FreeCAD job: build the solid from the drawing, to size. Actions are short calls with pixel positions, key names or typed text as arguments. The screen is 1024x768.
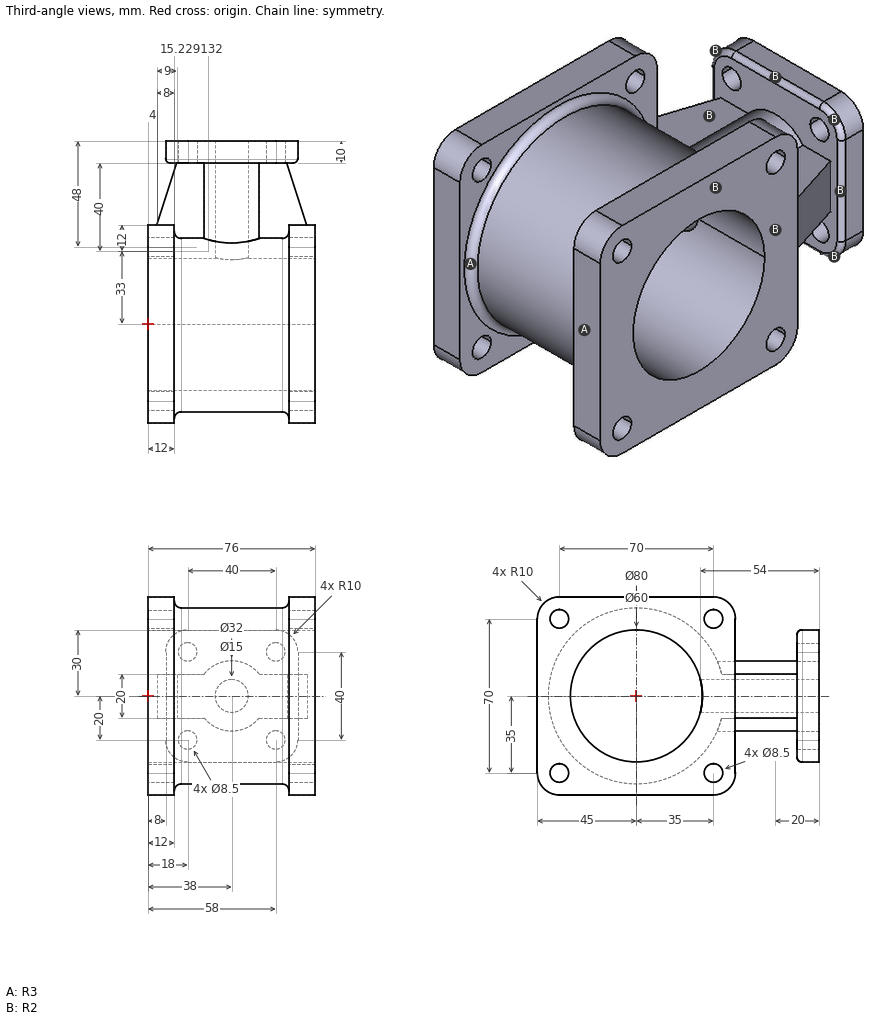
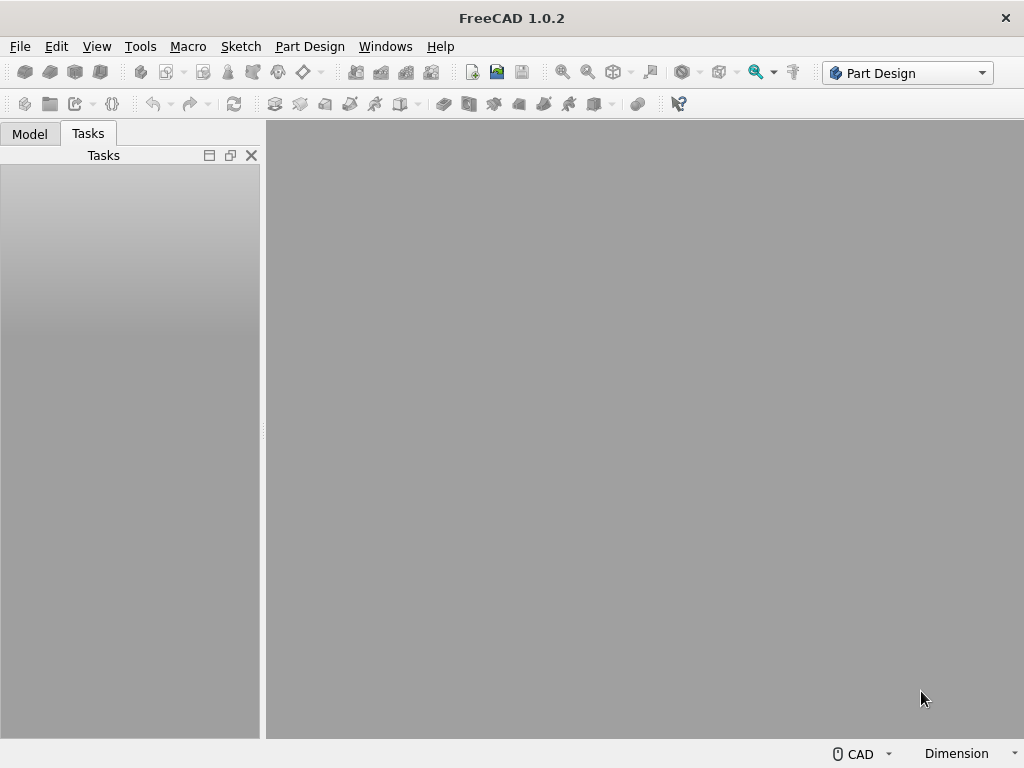
key(ctrl+n)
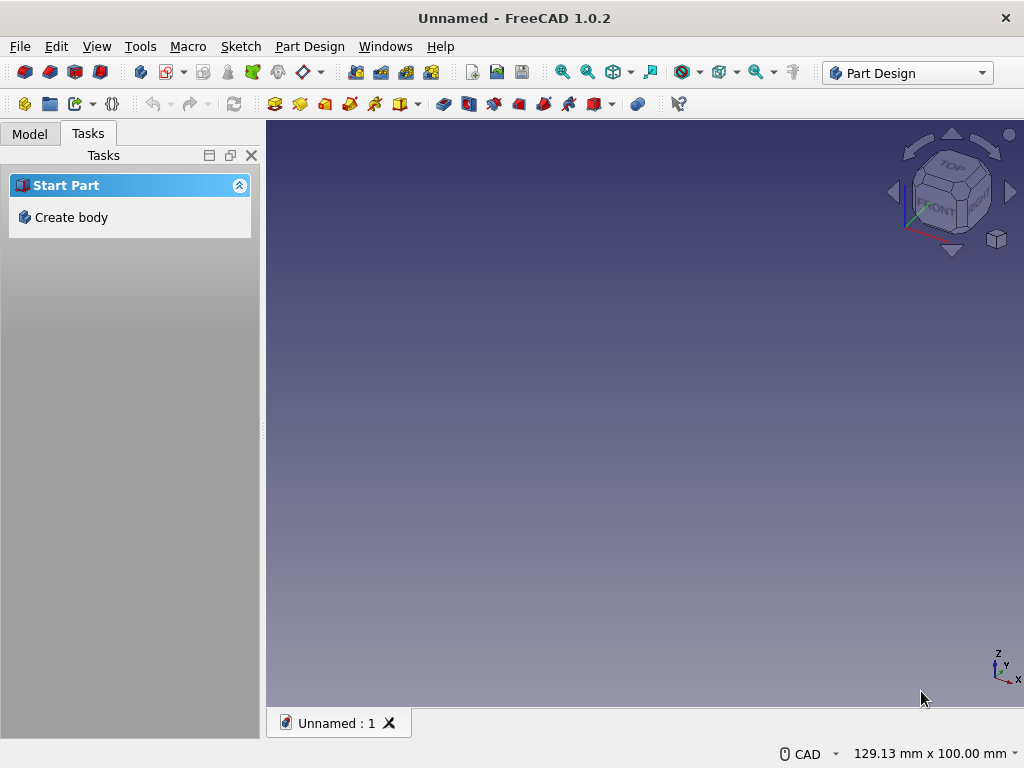
click(166, 72)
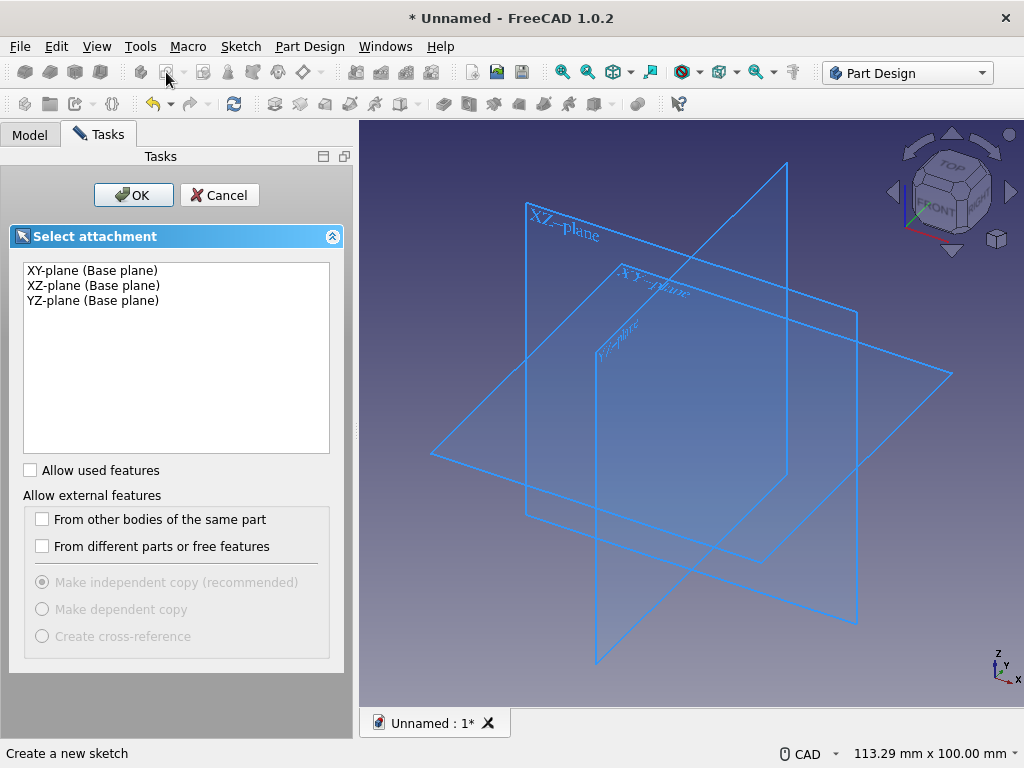
click(84, 300)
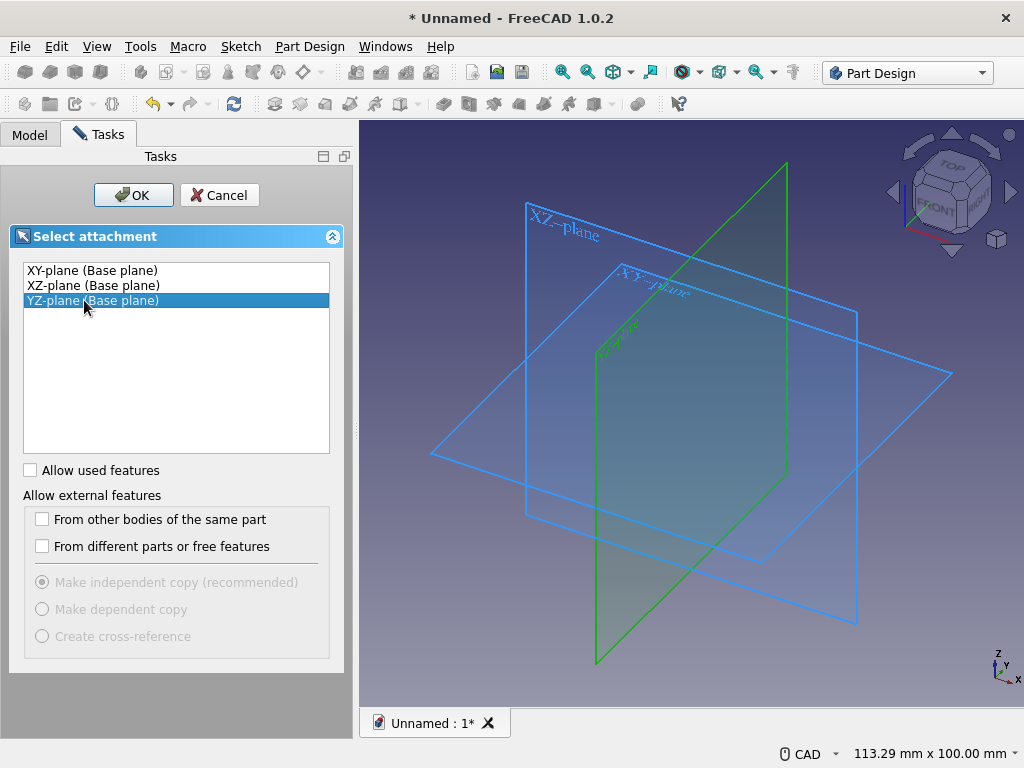
click(134, 195)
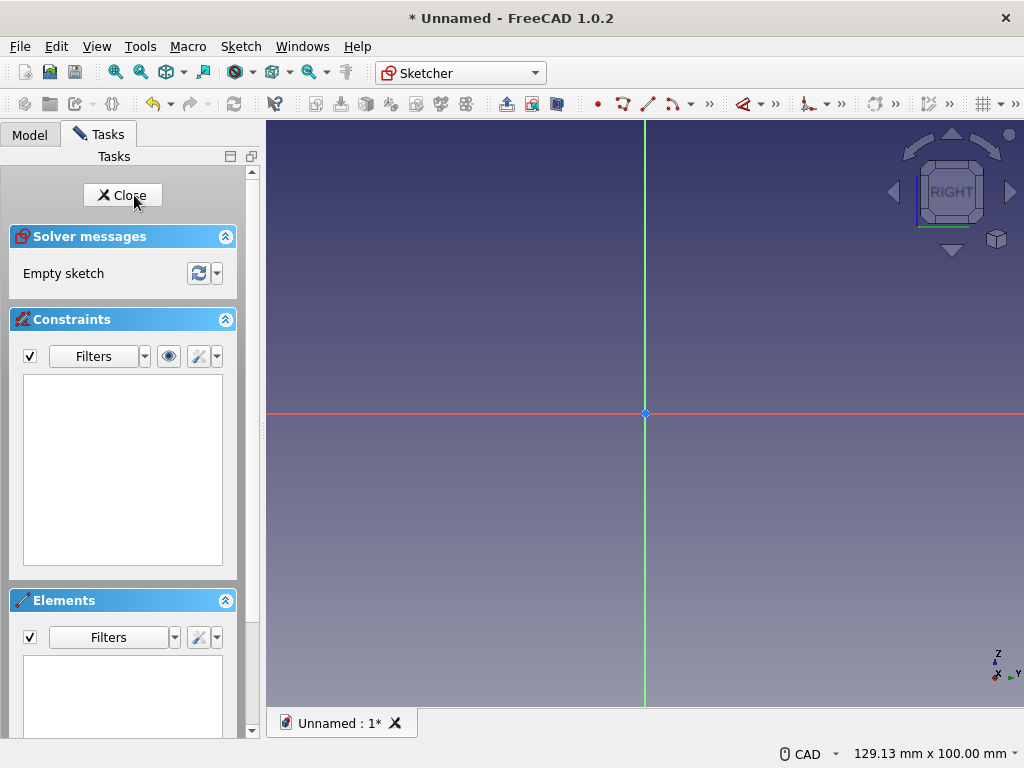
scroll(294, 413, down, 1)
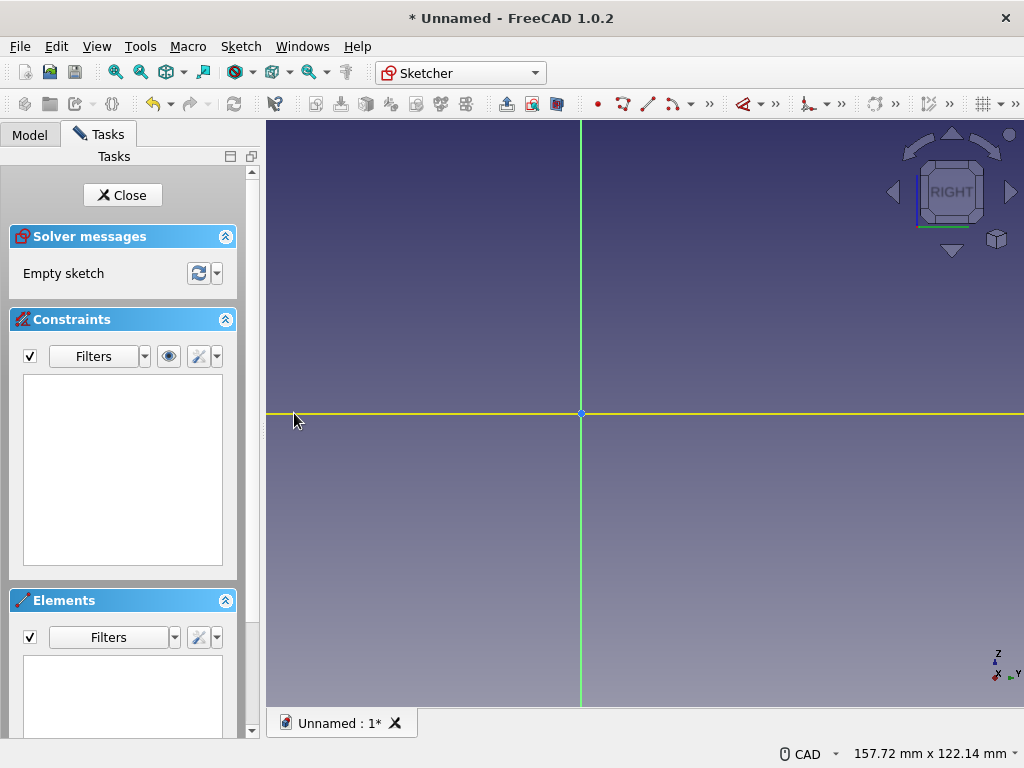
key(g)
key(c)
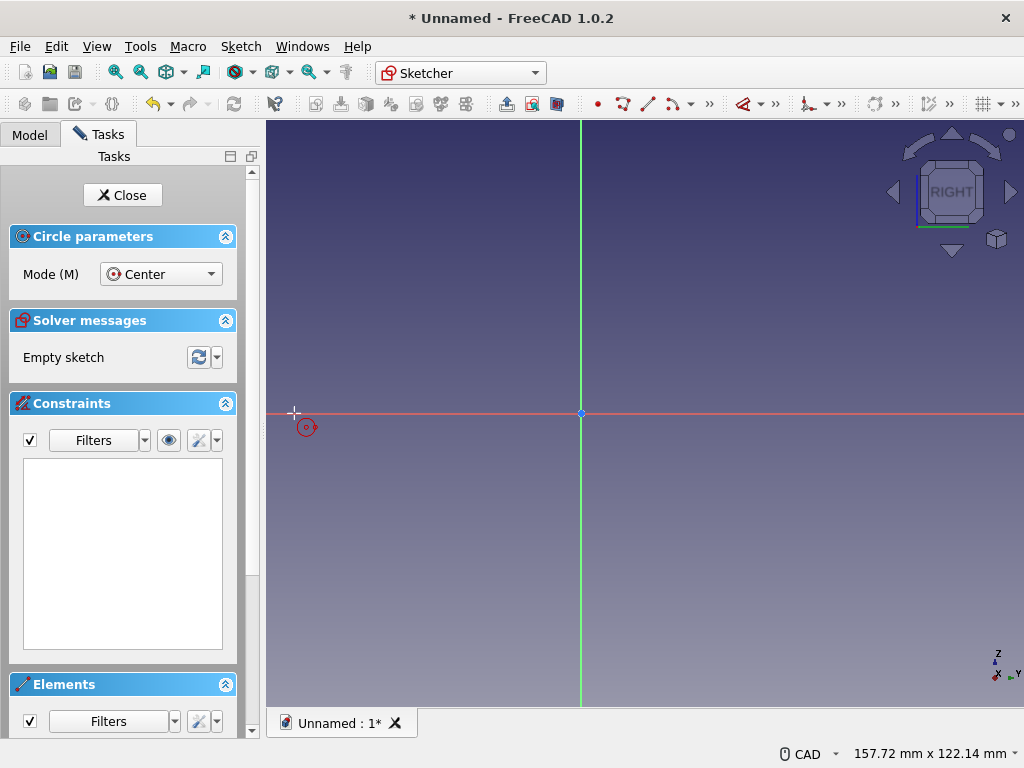
click(581, 414)
click(717, 278)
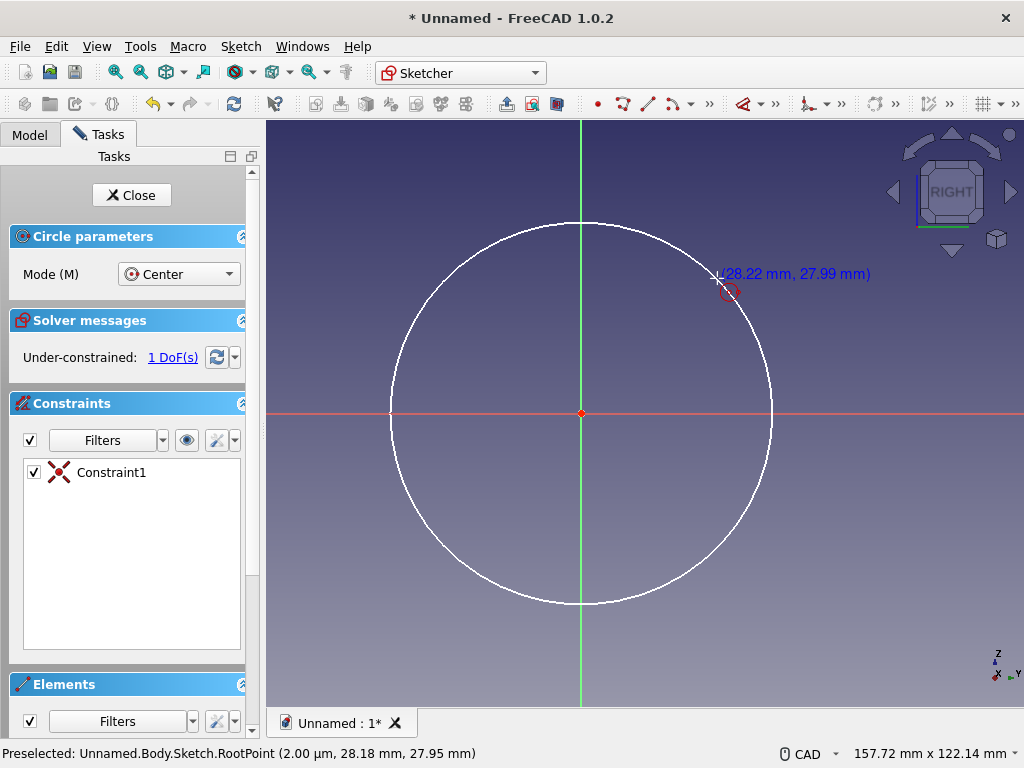
click(581, 414)
click(683, 312)
key(Escape)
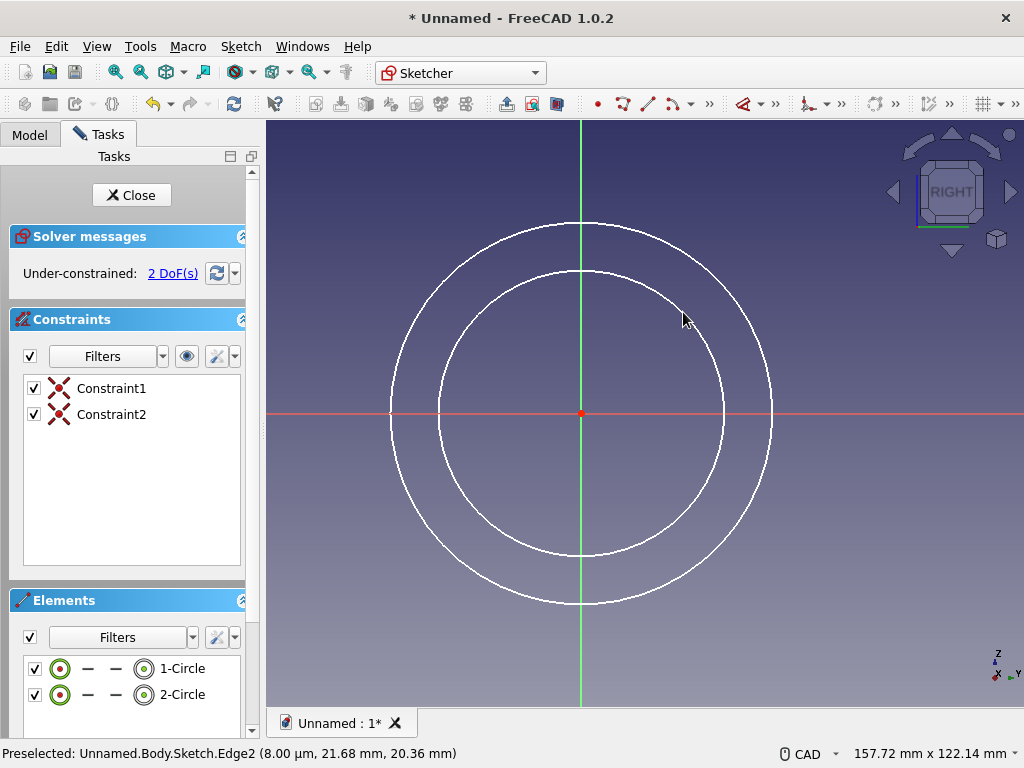
key(d)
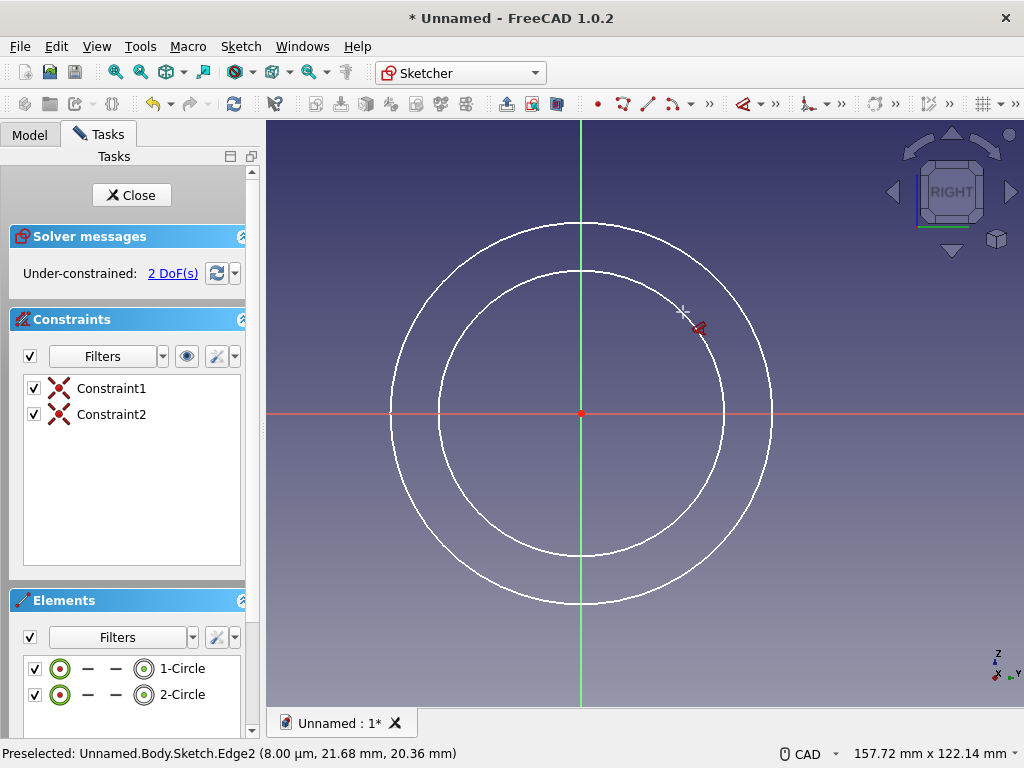
click(716, 278)
click(739, 255)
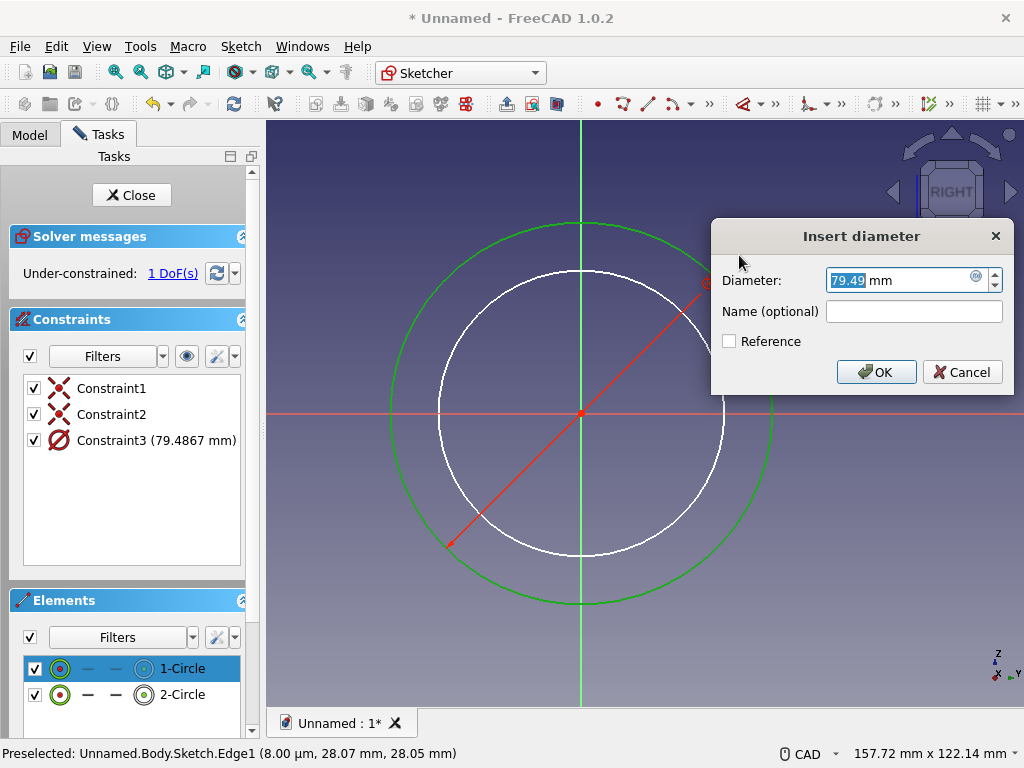
text(80)
key(Return)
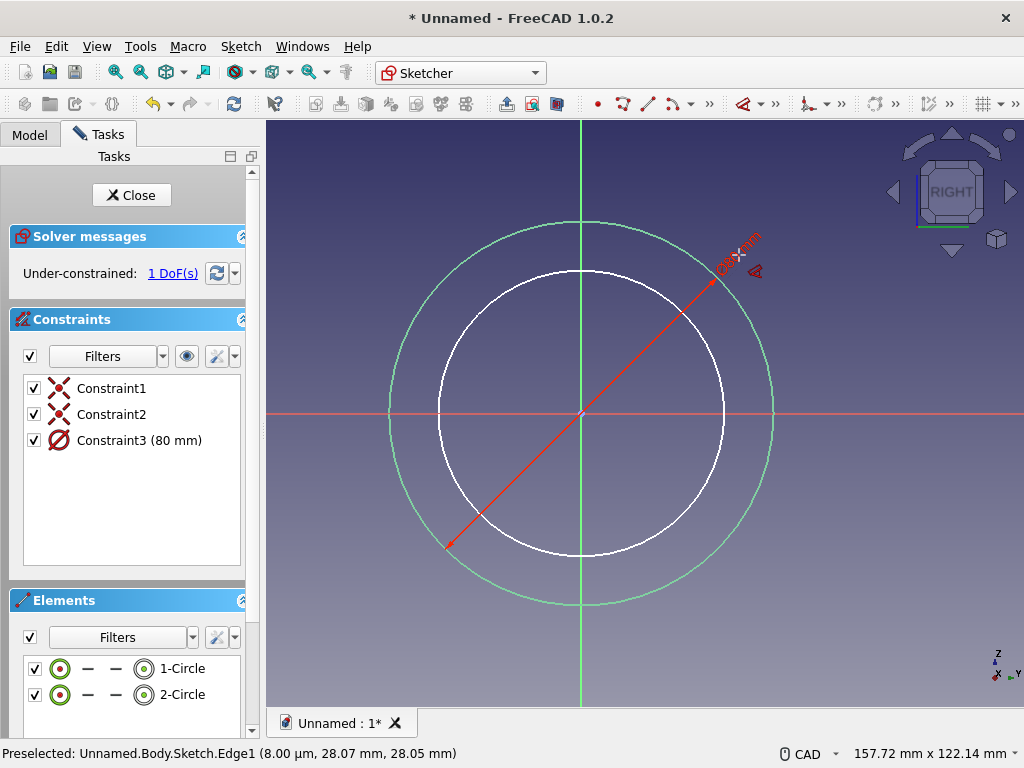
click(682, 312)
click(705, 289)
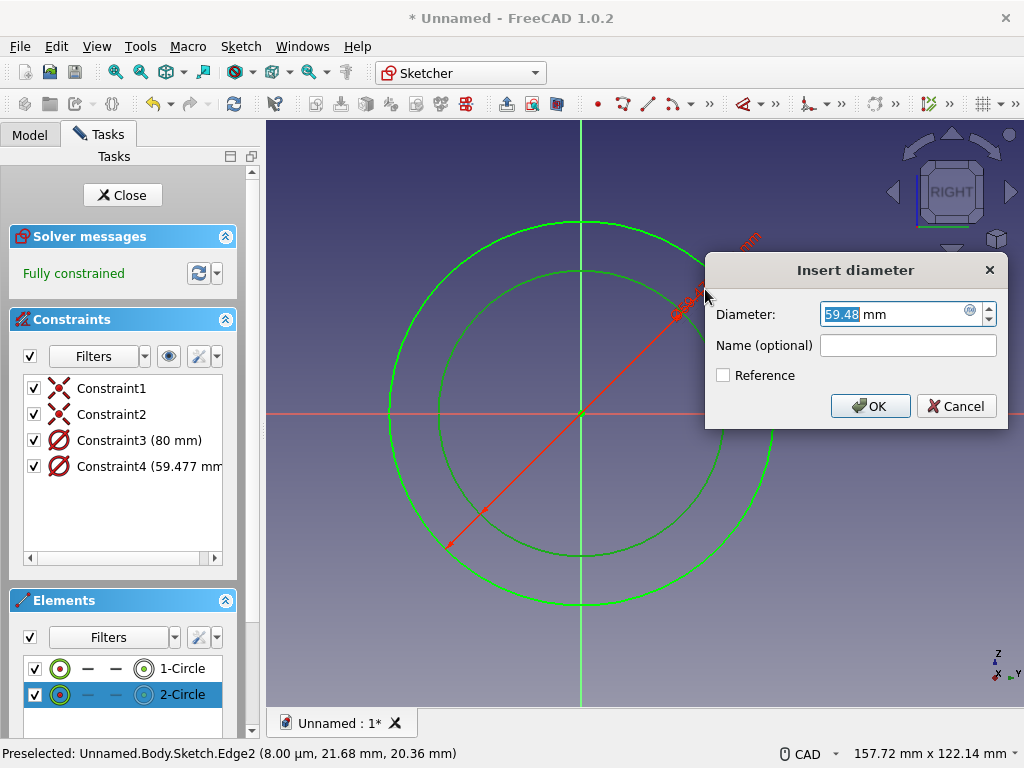
text(60)
key(Return)
key(Escape)